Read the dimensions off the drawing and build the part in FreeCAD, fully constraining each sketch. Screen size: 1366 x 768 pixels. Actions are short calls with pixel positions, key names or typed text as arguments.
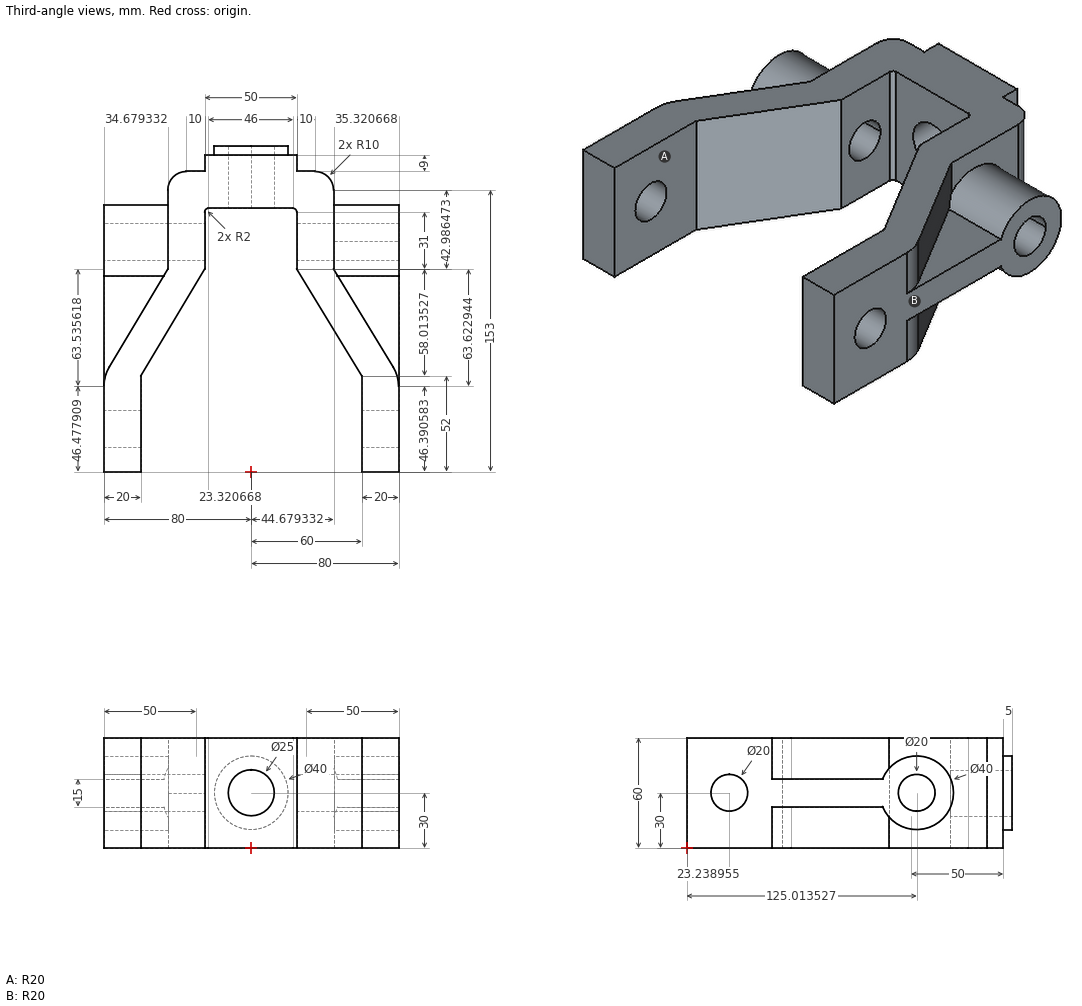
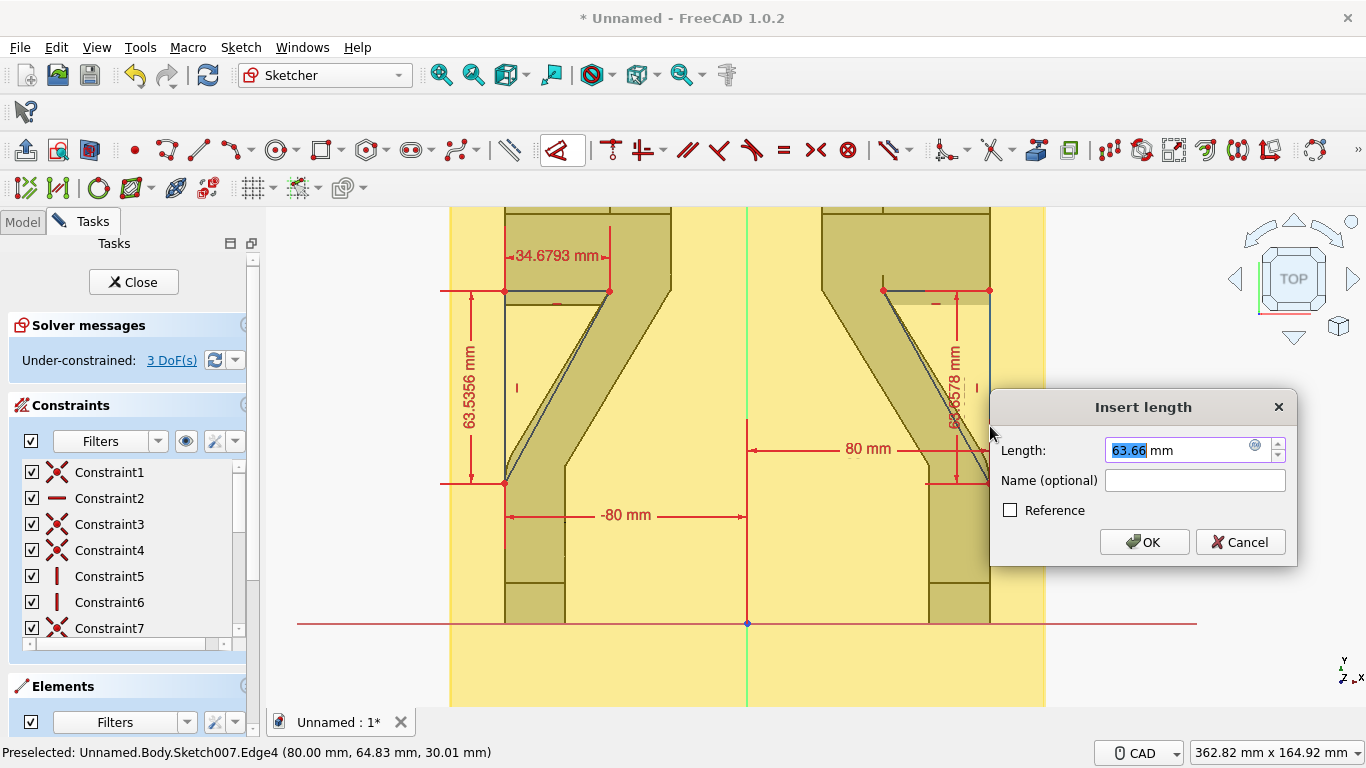
text(63.622944)
key(Return)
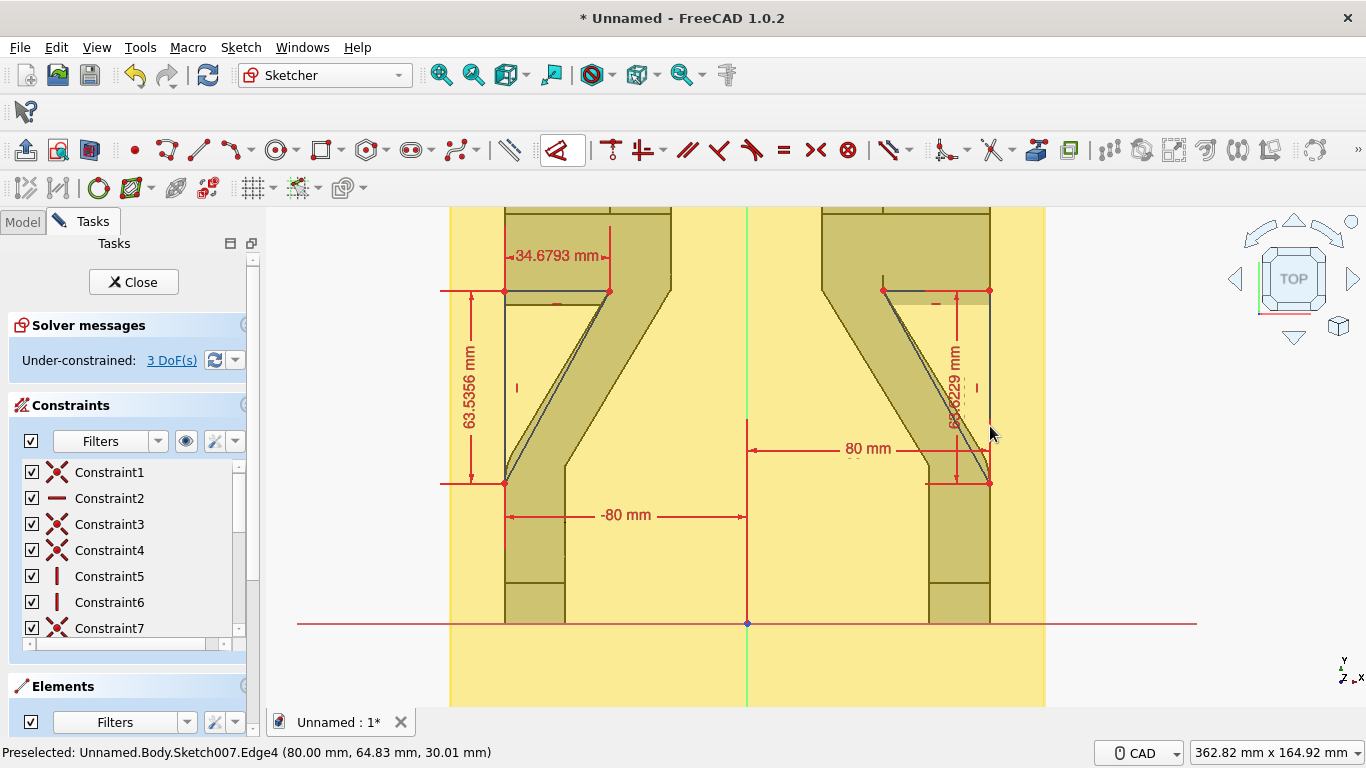
click(958, 291)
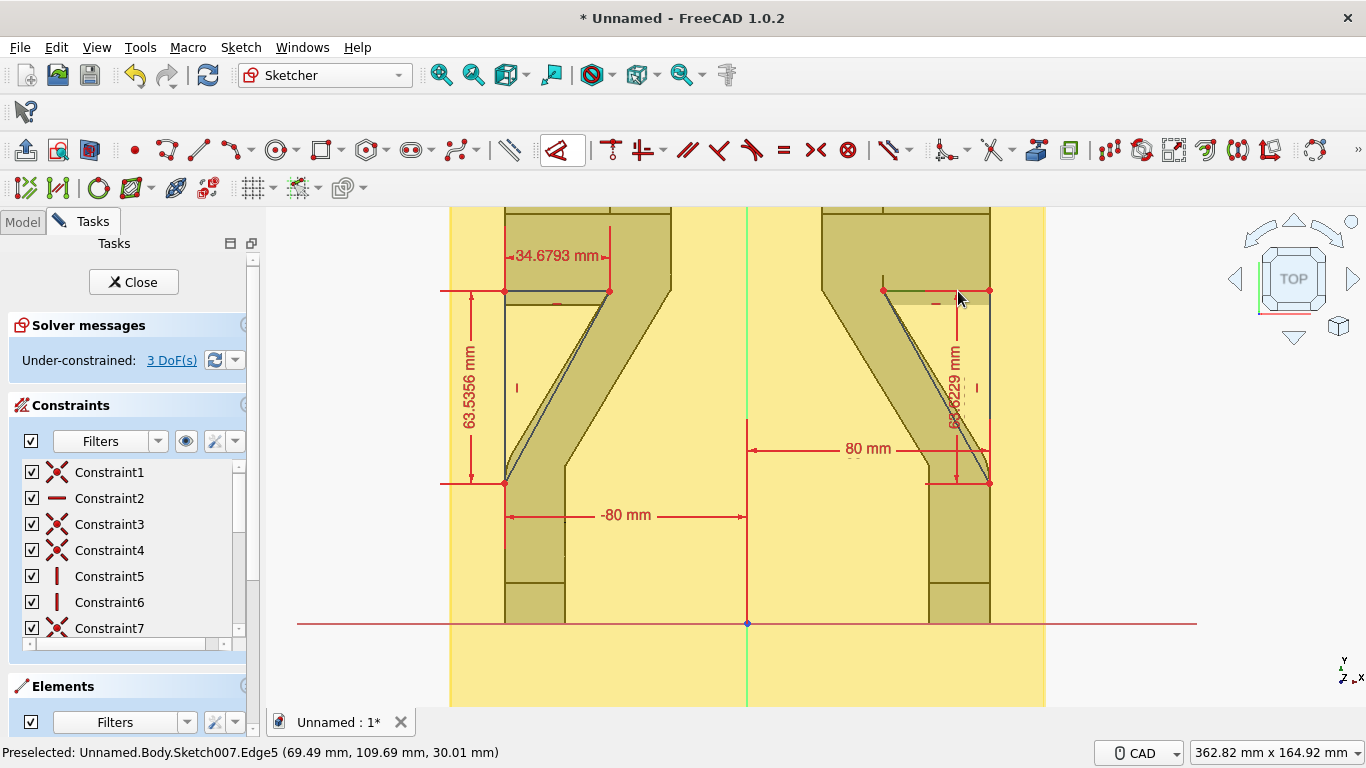
key(l)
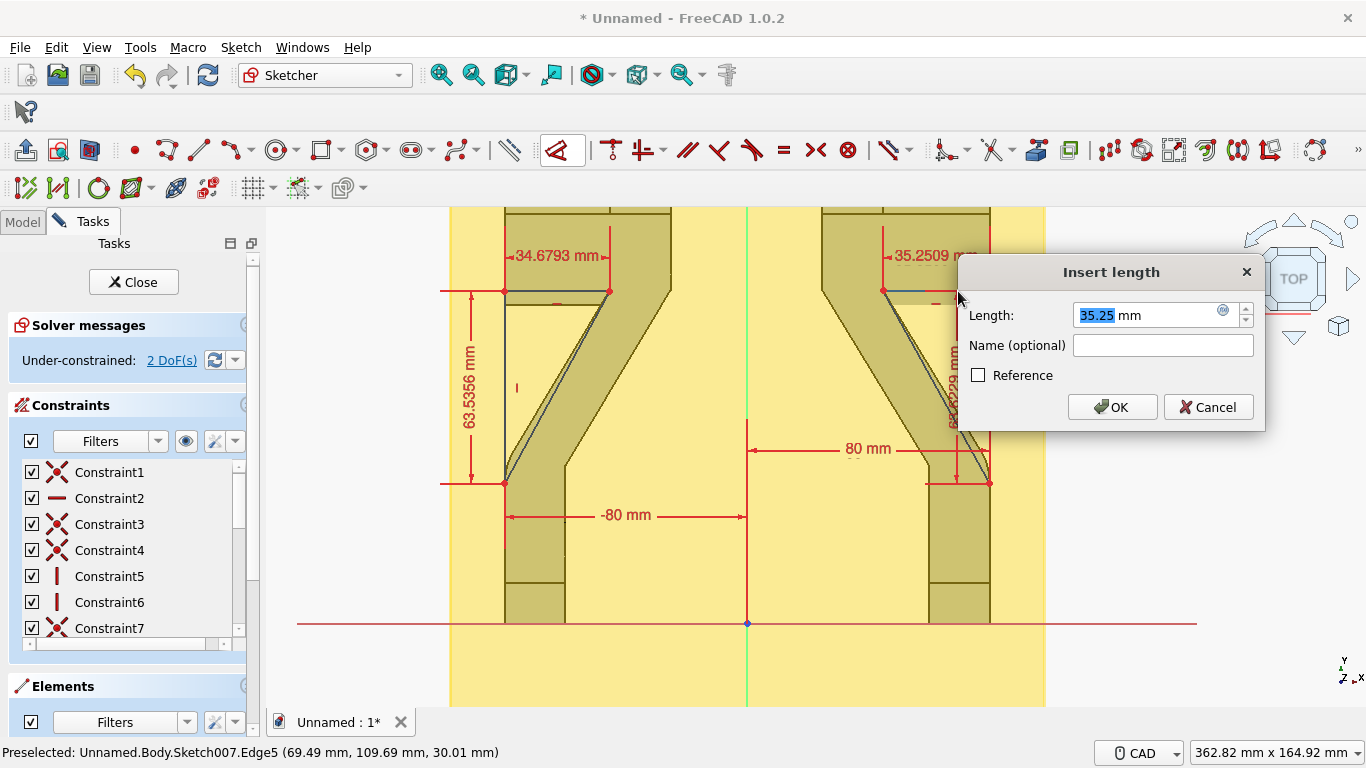
text(35.320668)
key(Return)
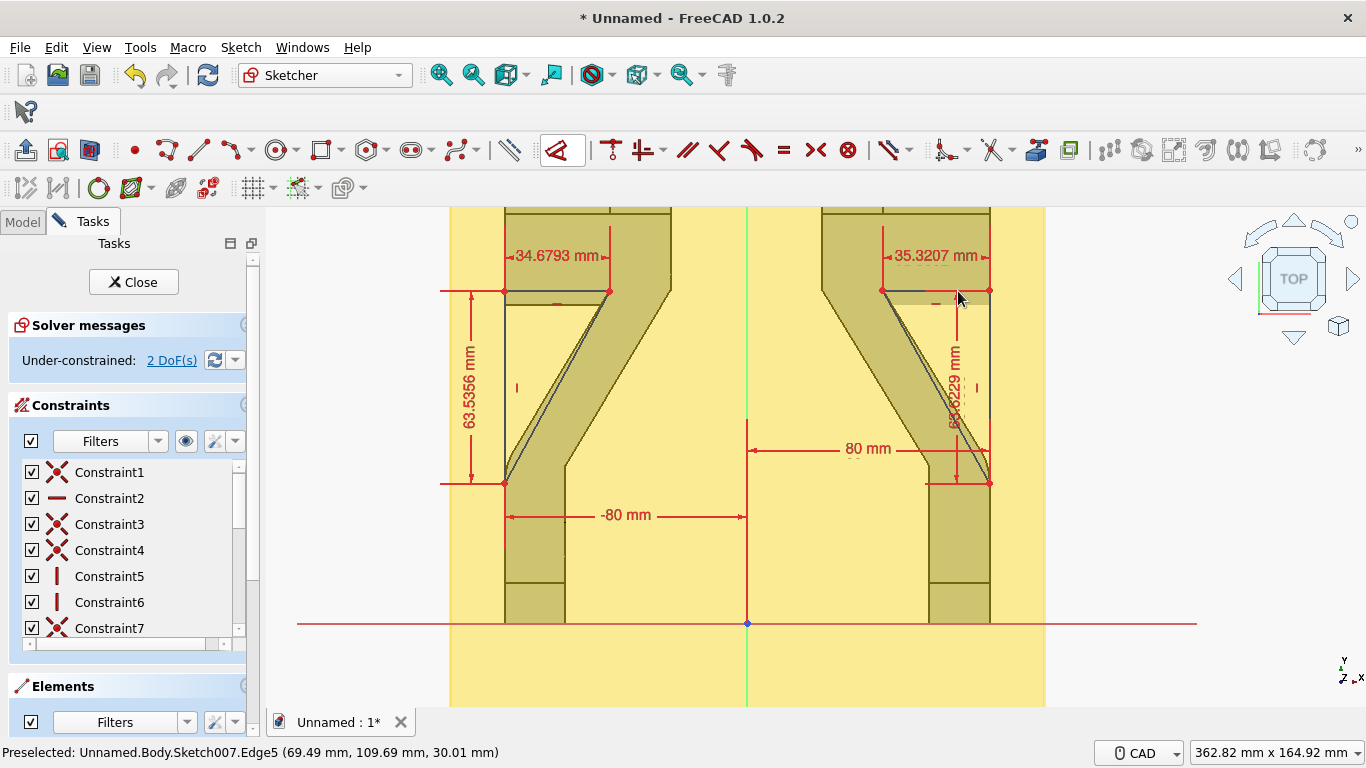
click(505, 484)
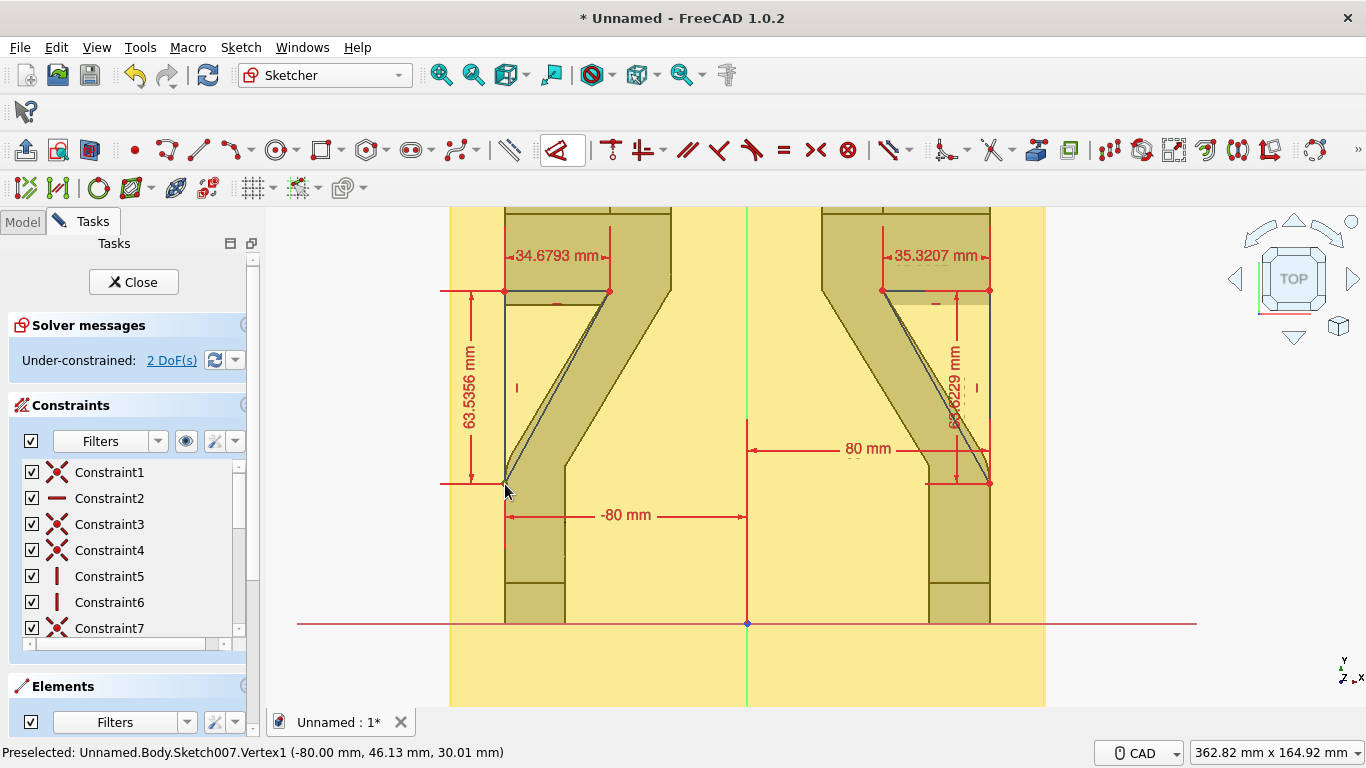
click(580, 150)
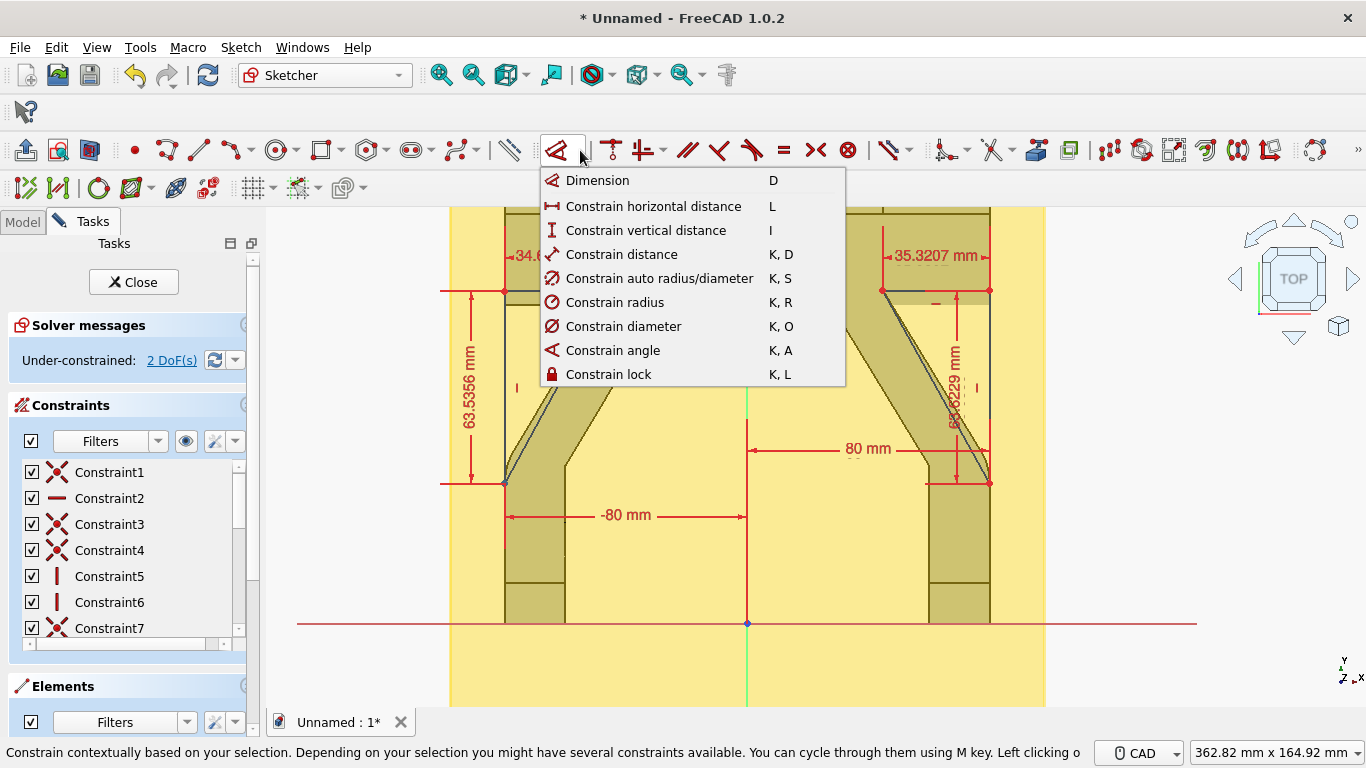
click(693, 230)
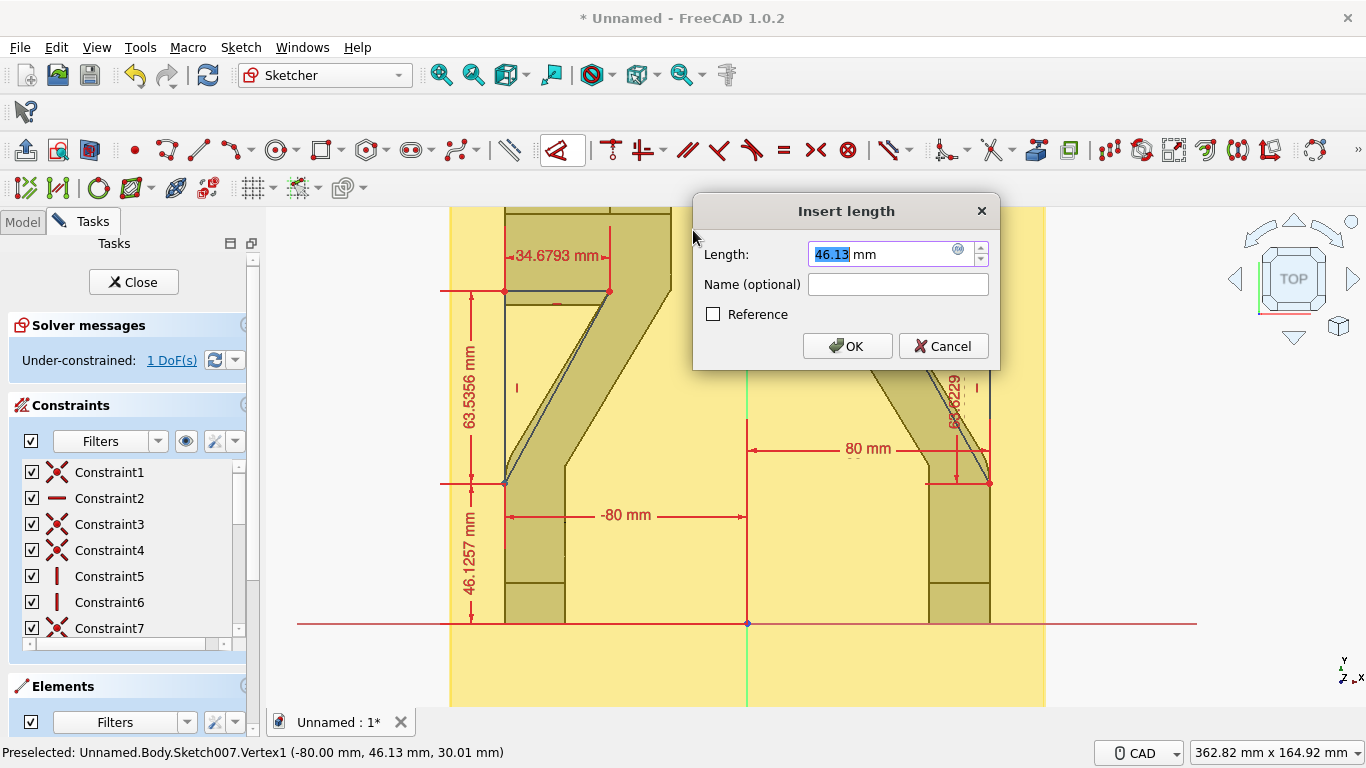
text(46.477909)
key(Return)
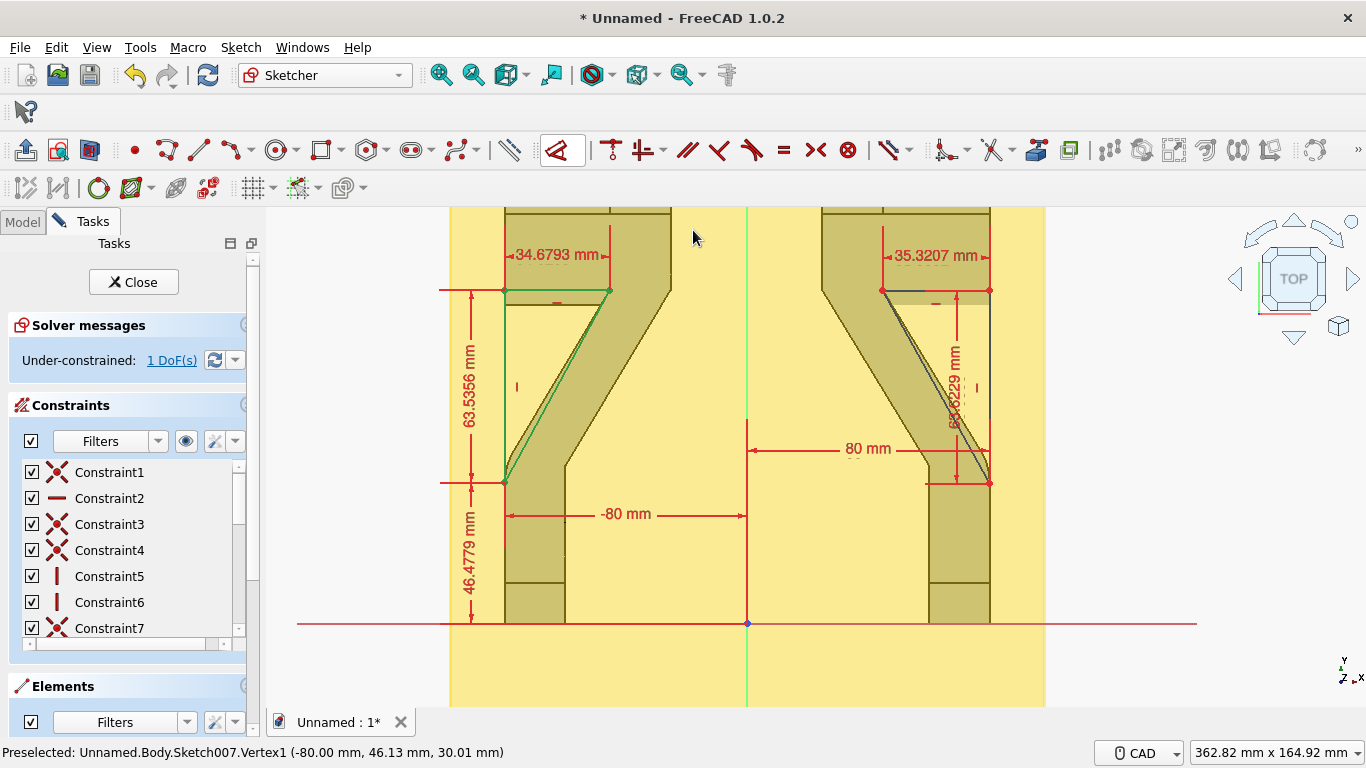
click(990, 484)